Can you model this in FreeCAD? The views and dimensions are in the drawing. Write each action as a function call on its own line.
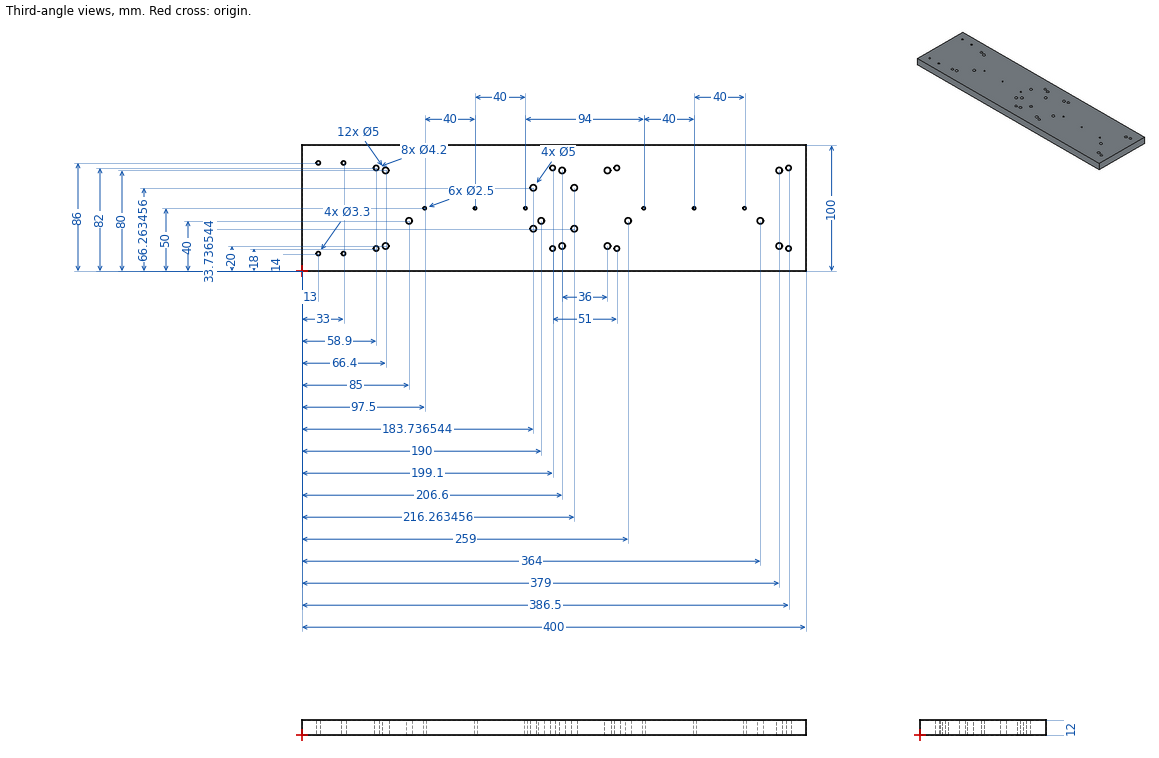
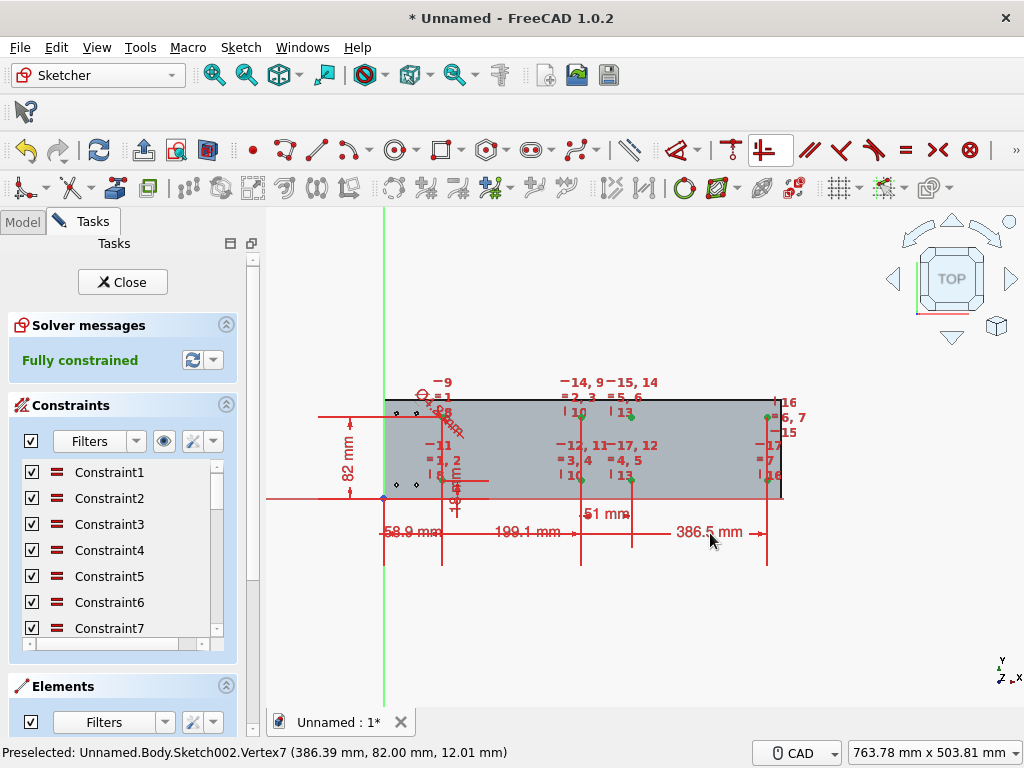
click(123, 282)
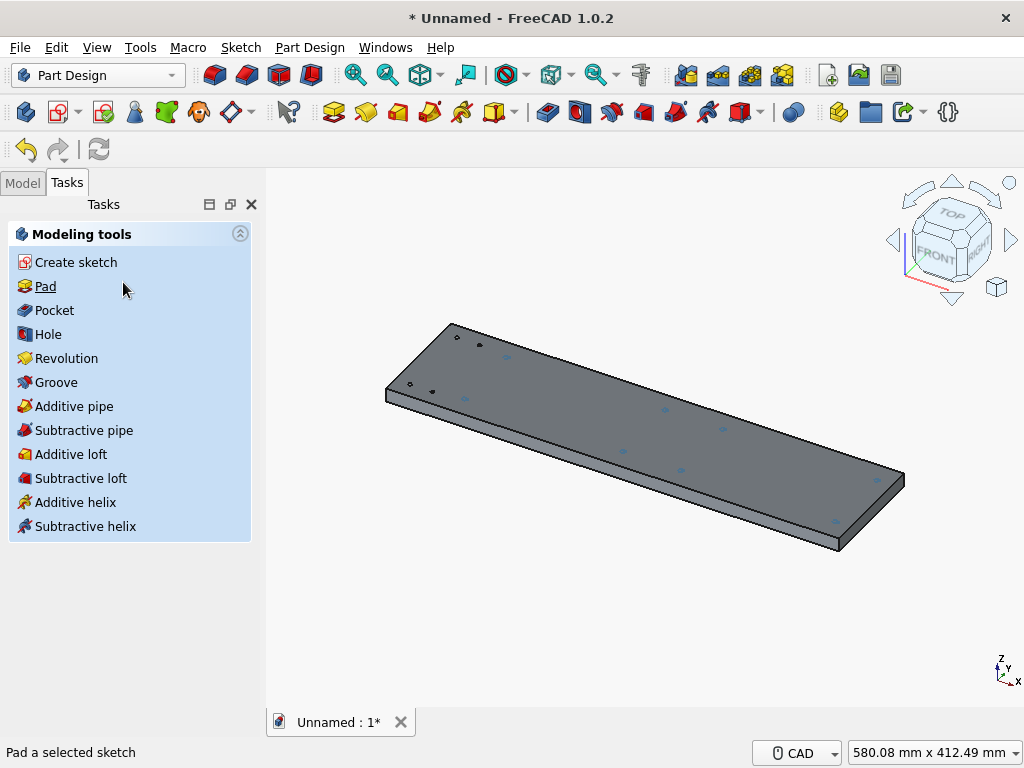
click(548, 112)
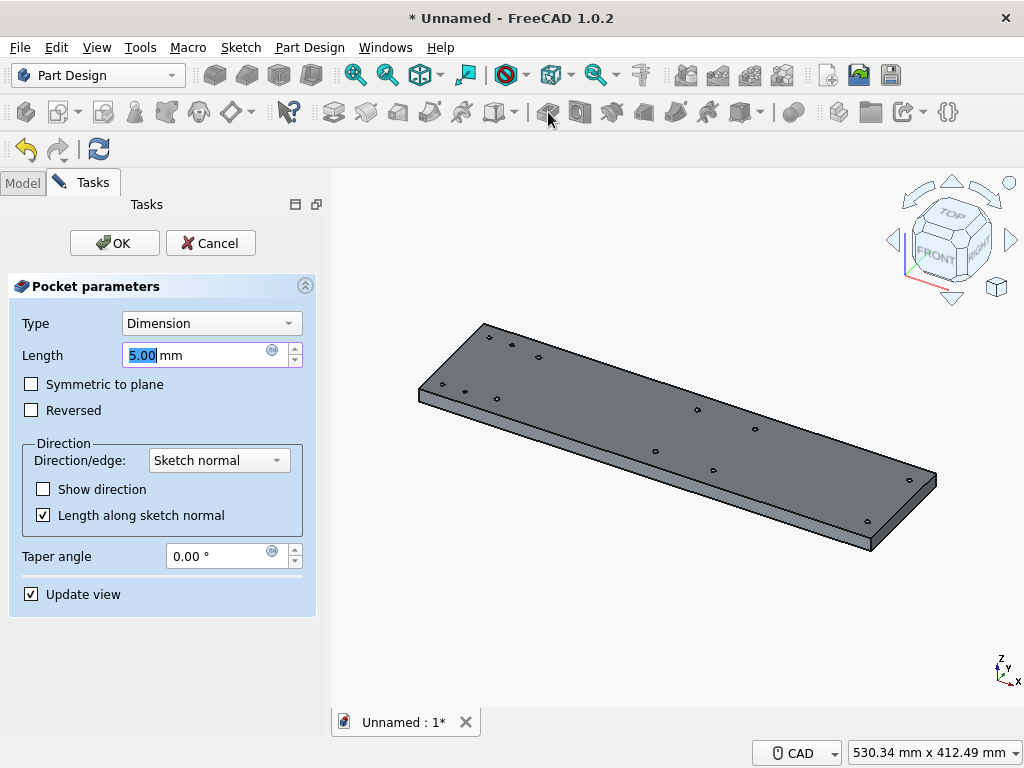
click(212, 324)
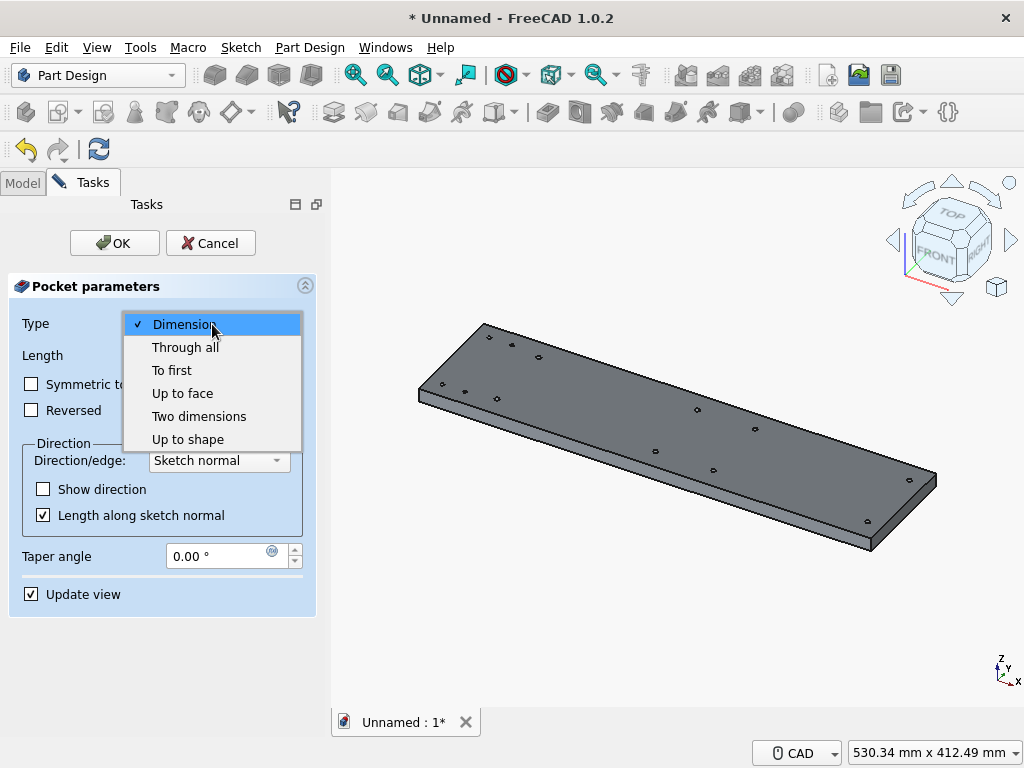
click(212, 348)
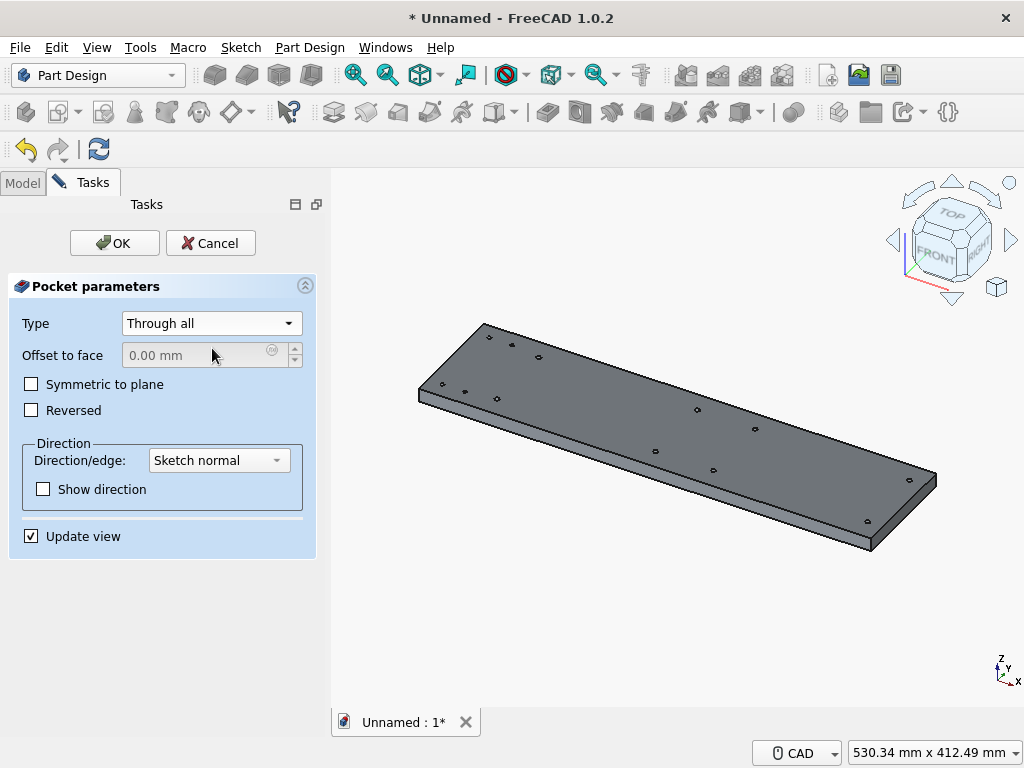
click(115, 243)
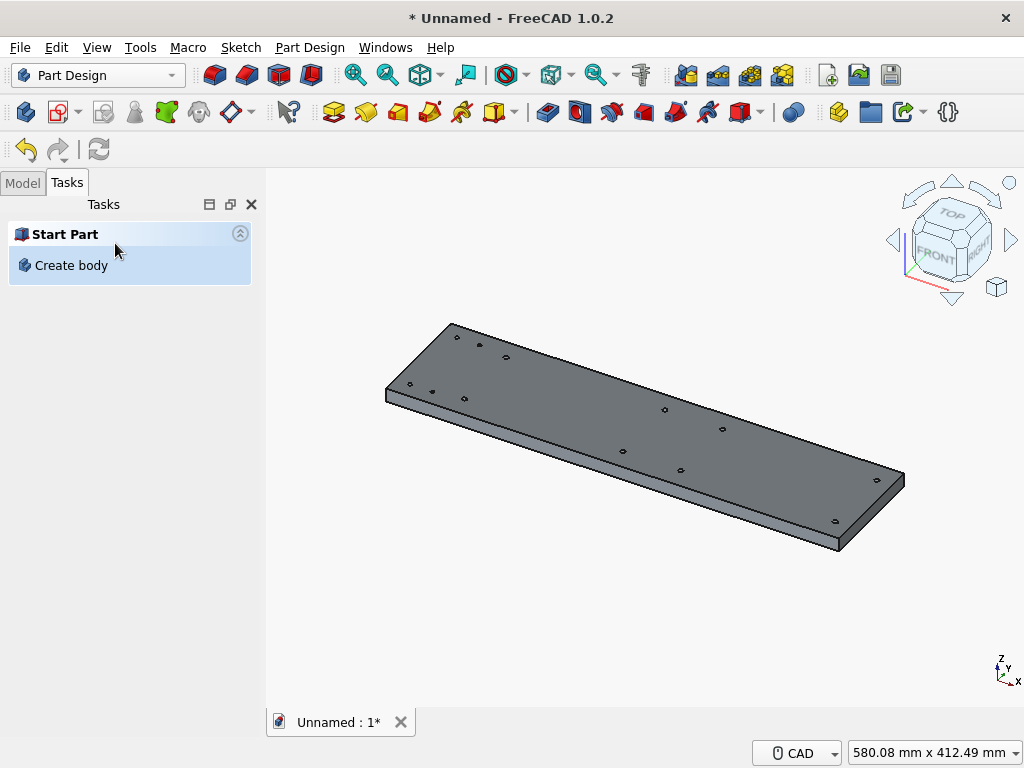
click(774, 473)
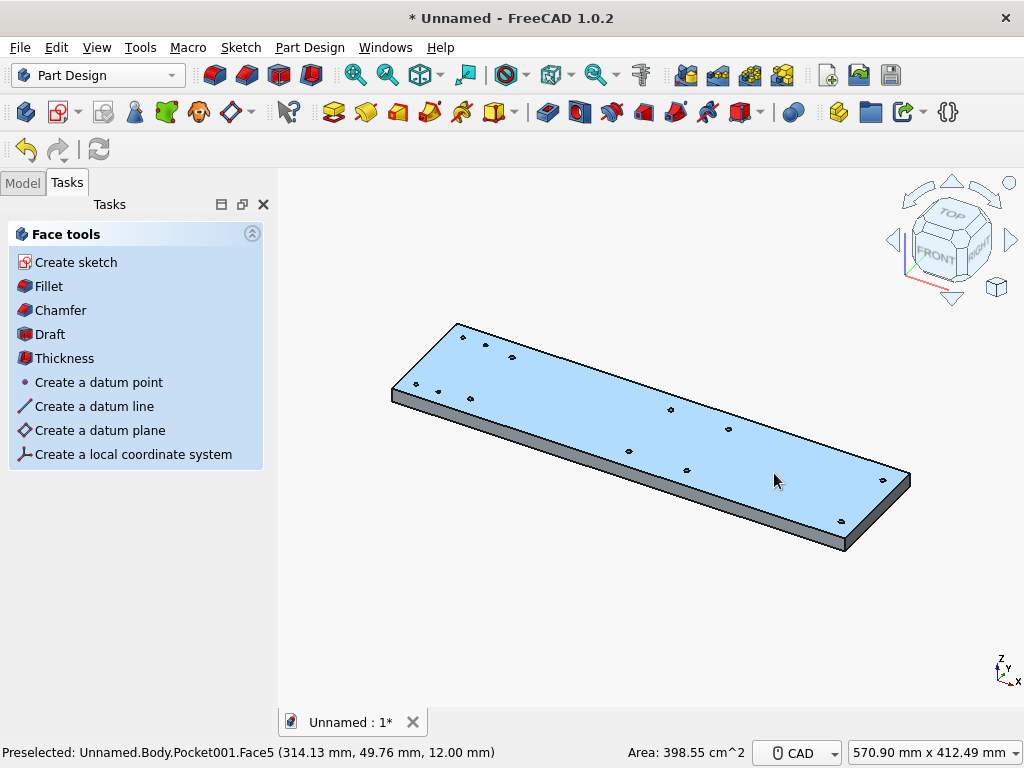
click(58, 112)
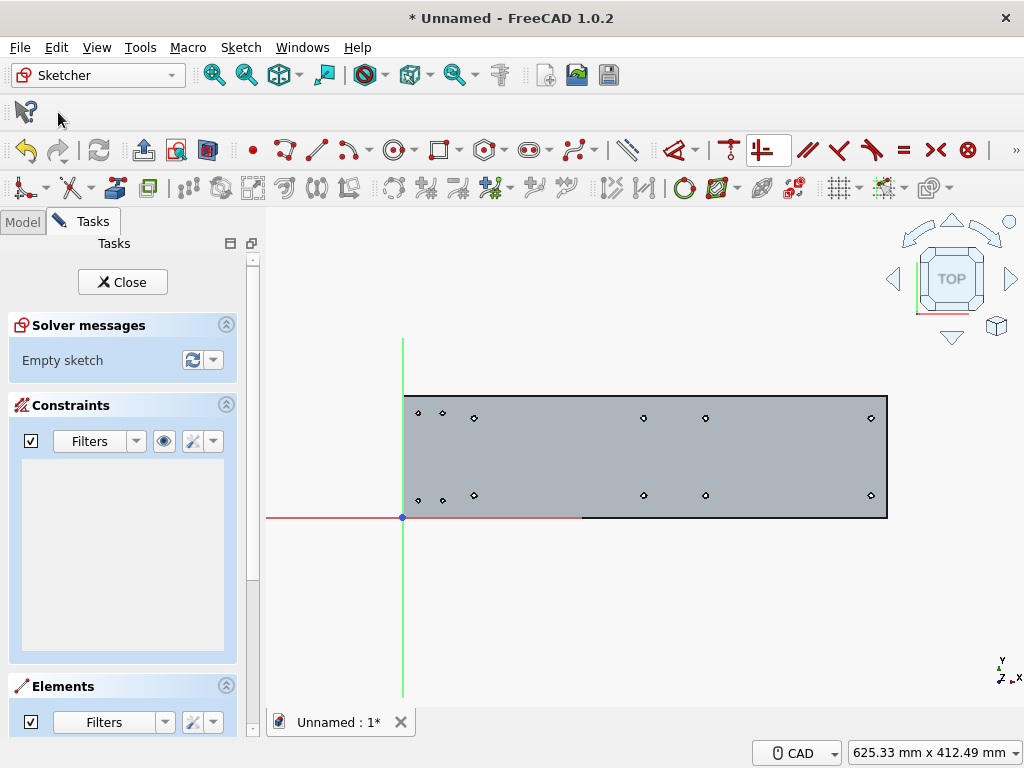
scroll(318, 409, down, 1)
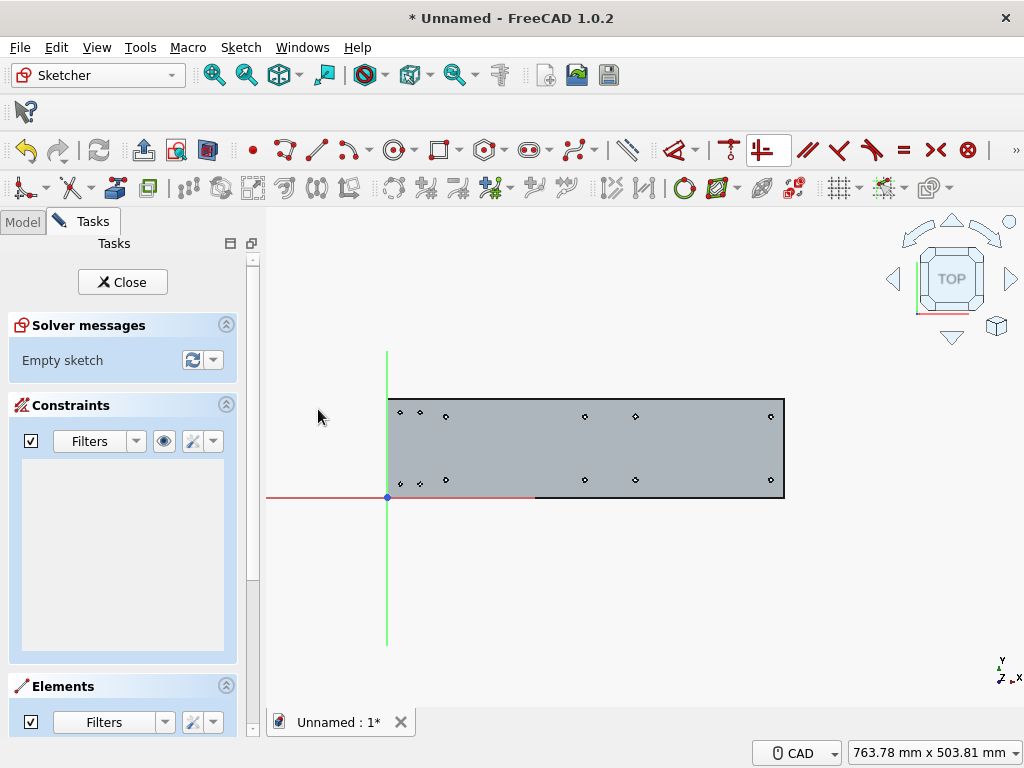
click(394, 150)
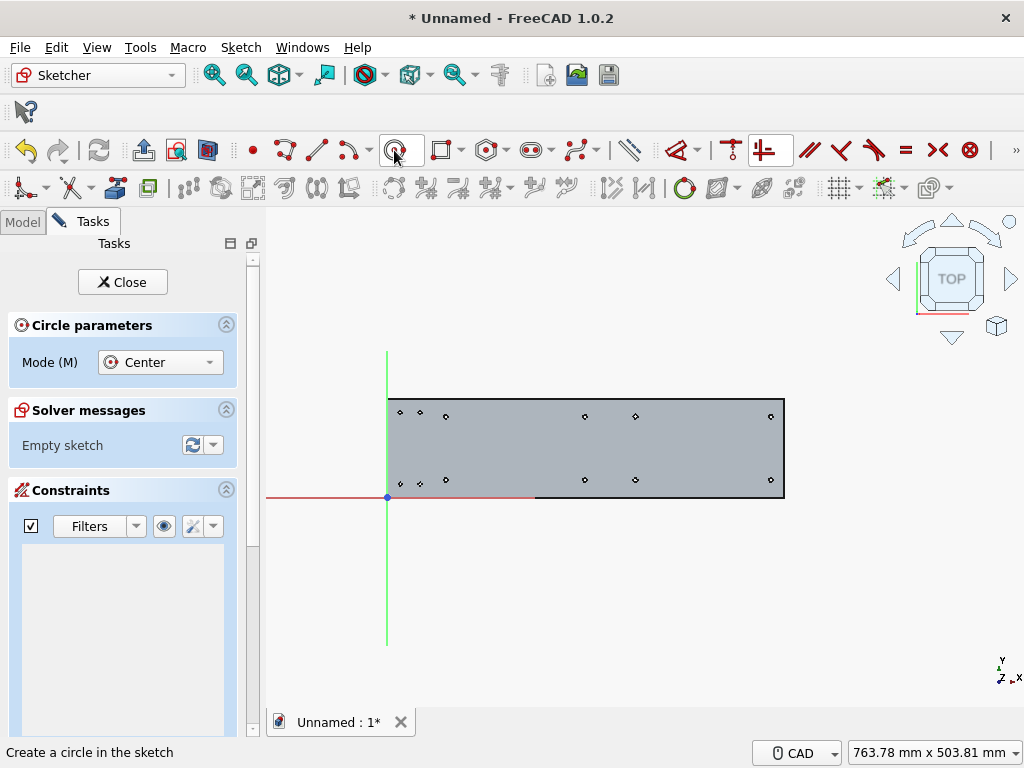
scroll(453, 419, up, 12)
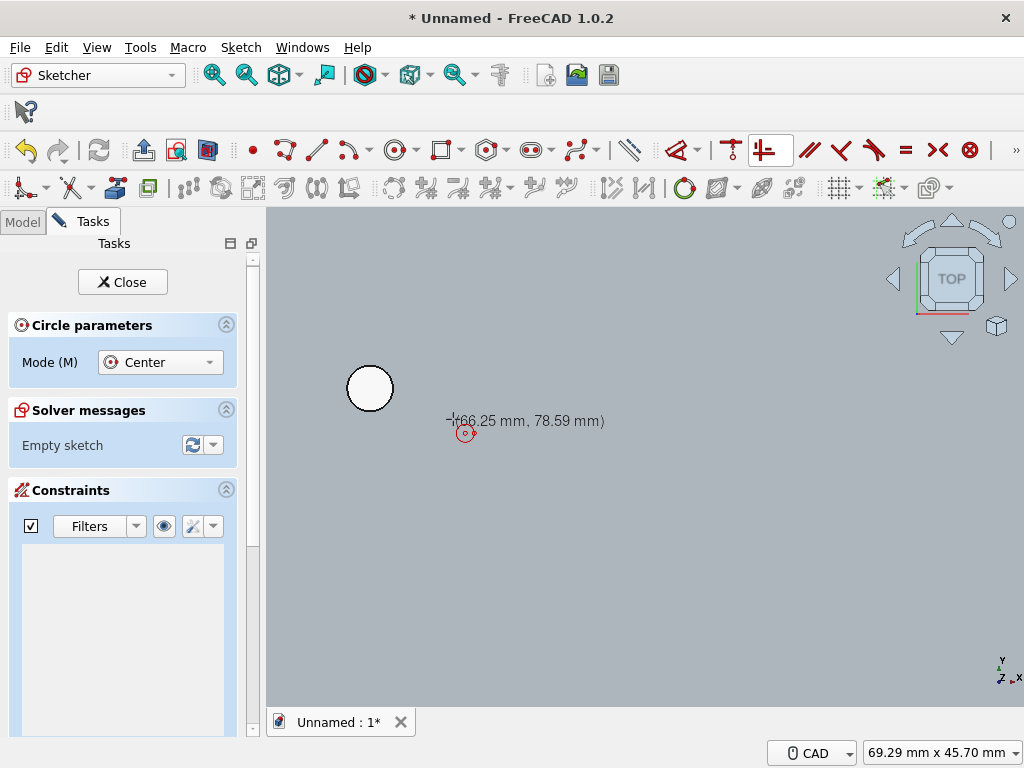
scroll(453, 419, down, 12)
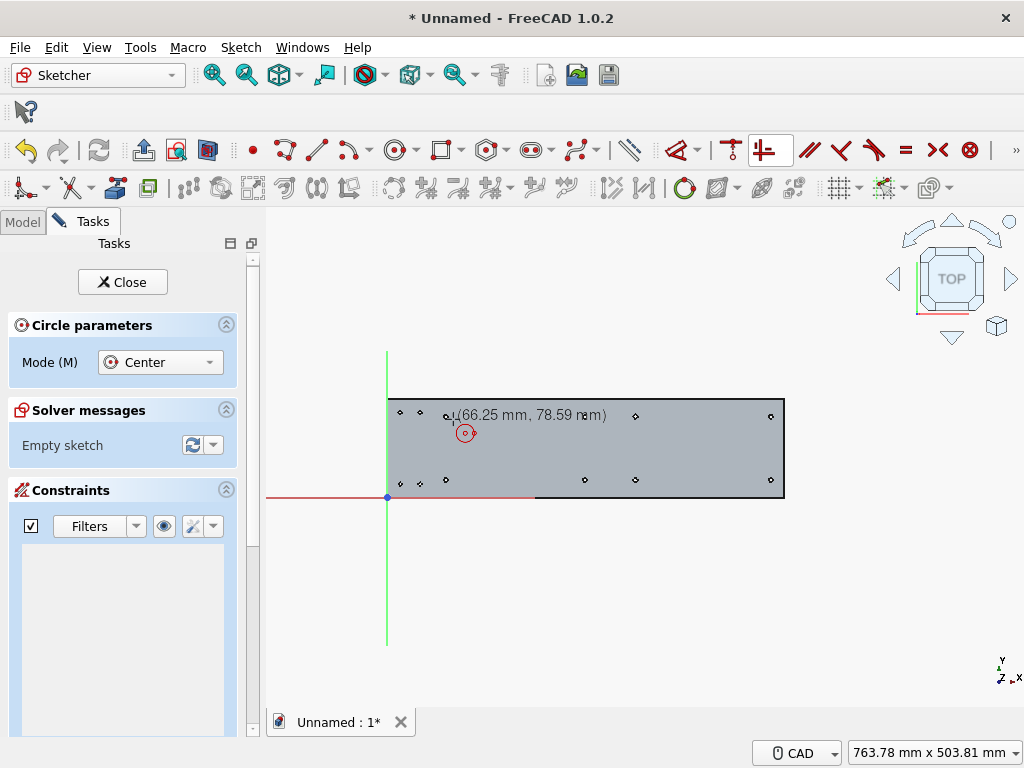
click(453, 419)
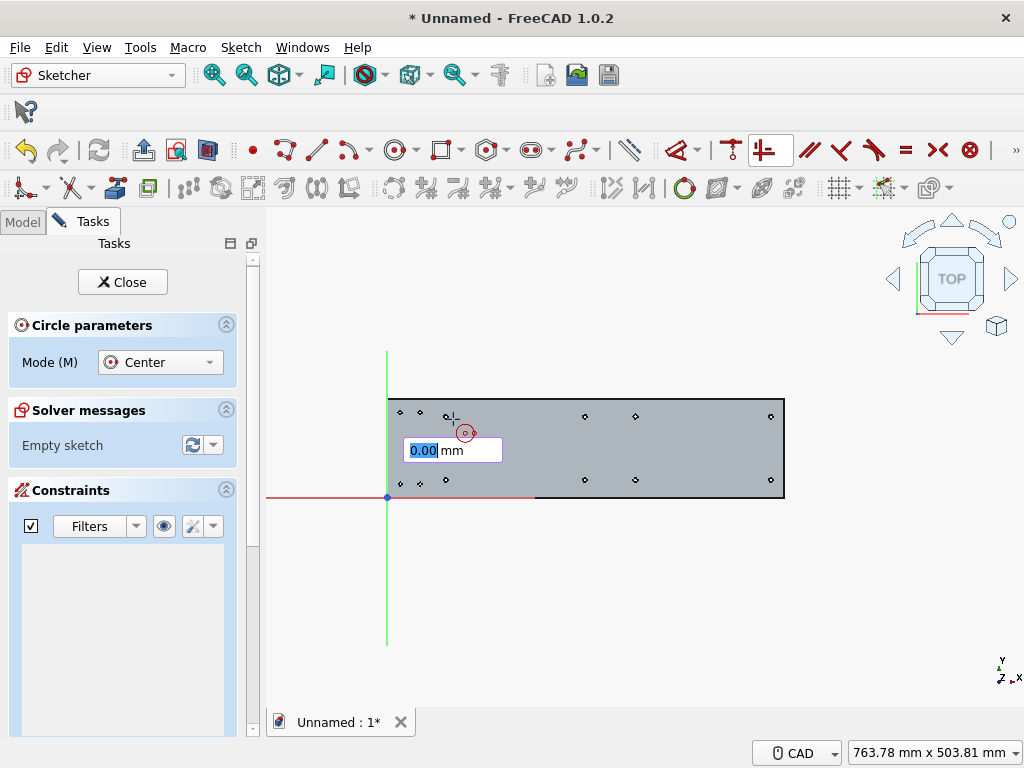
scroll(455, 417, up, 10)